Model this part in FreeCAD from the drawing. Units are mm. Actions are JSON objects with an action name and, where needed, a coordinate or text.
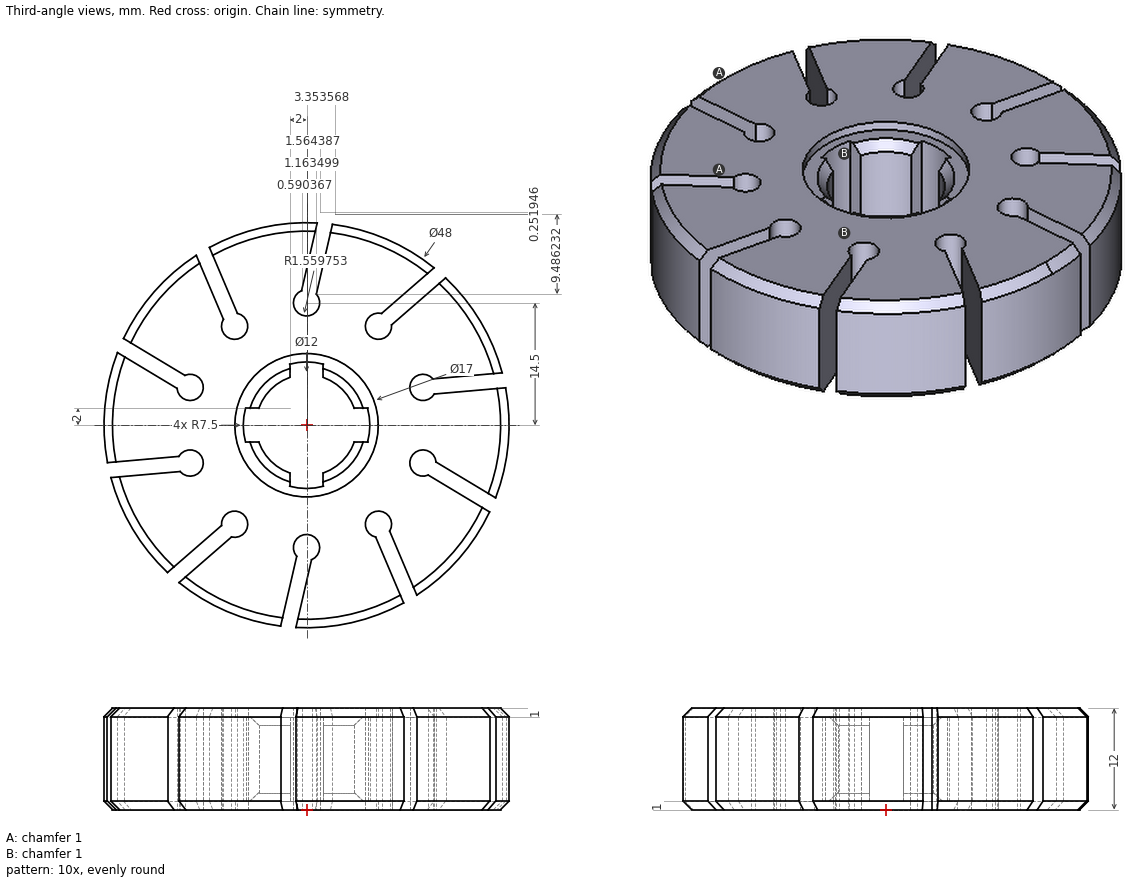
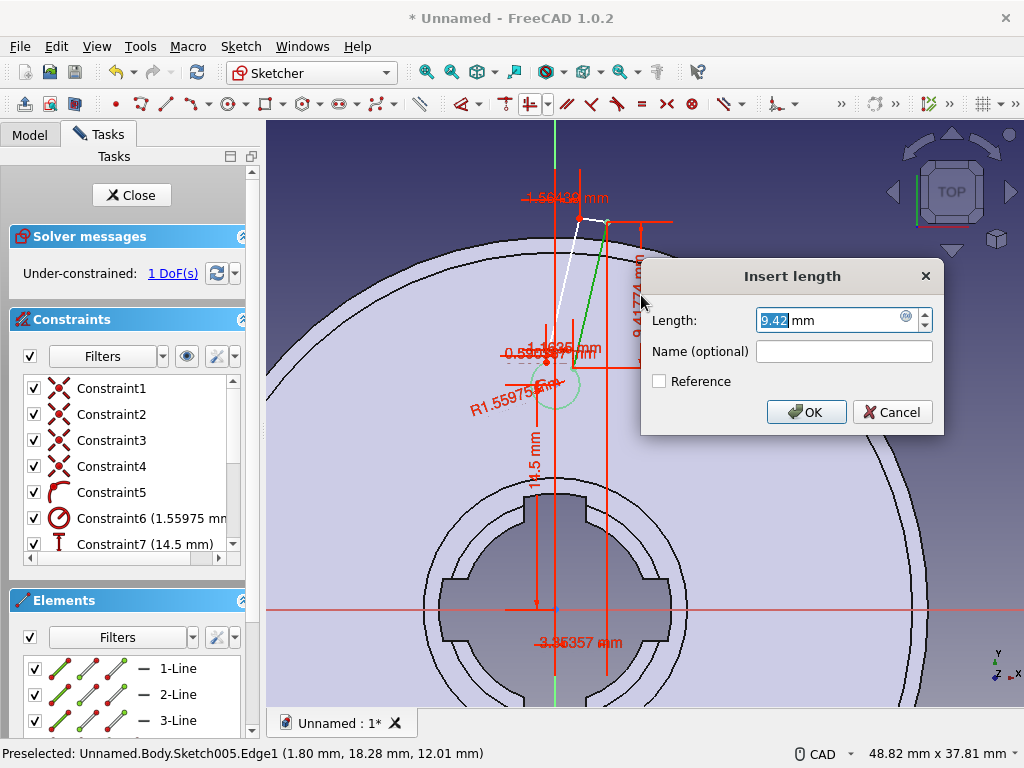
{"action": "type", "text": "9.486232"}
{"action": "key", "text": "Return"}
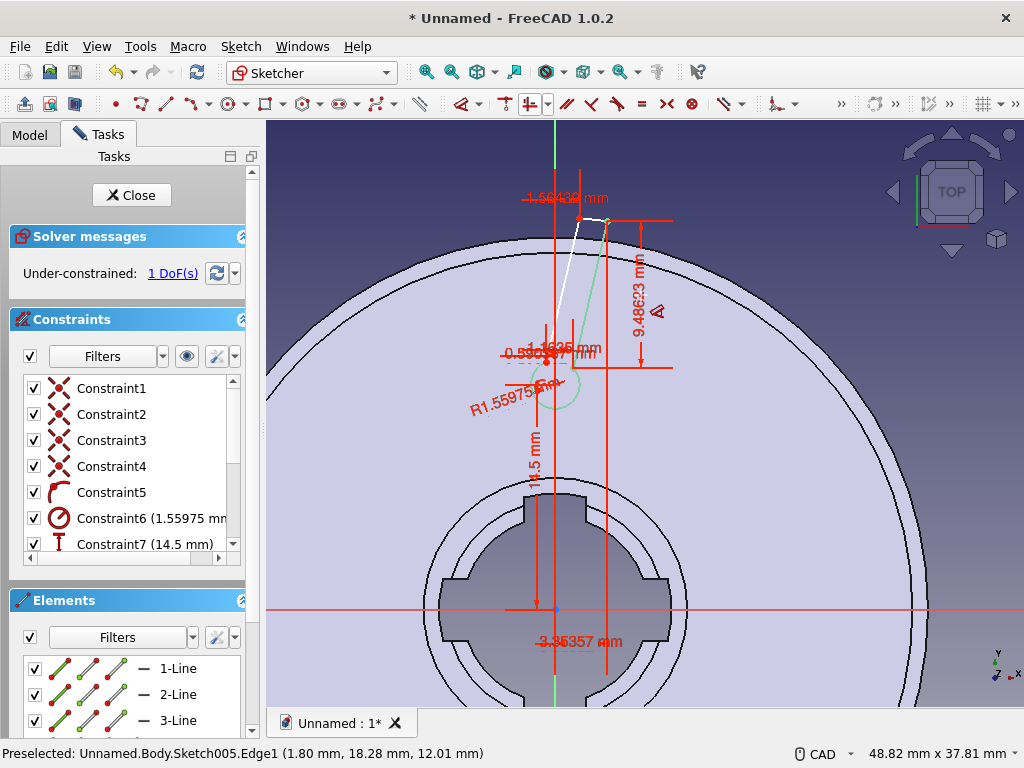
{"action": "scroll", "coordinate": [596, 220], "scroll_direction": "up", "scroll_amount": 12}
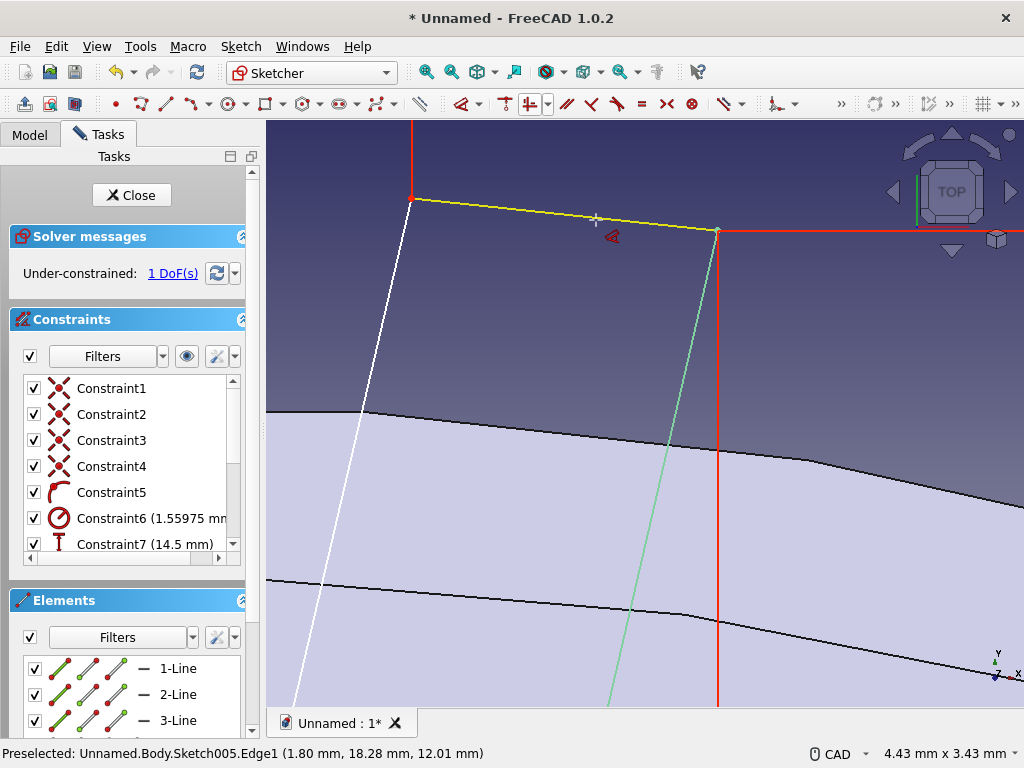
{"action": "left_click", "coordinate": [595, 218]}
{"action": "left_click", "coordinate": [752, 215]}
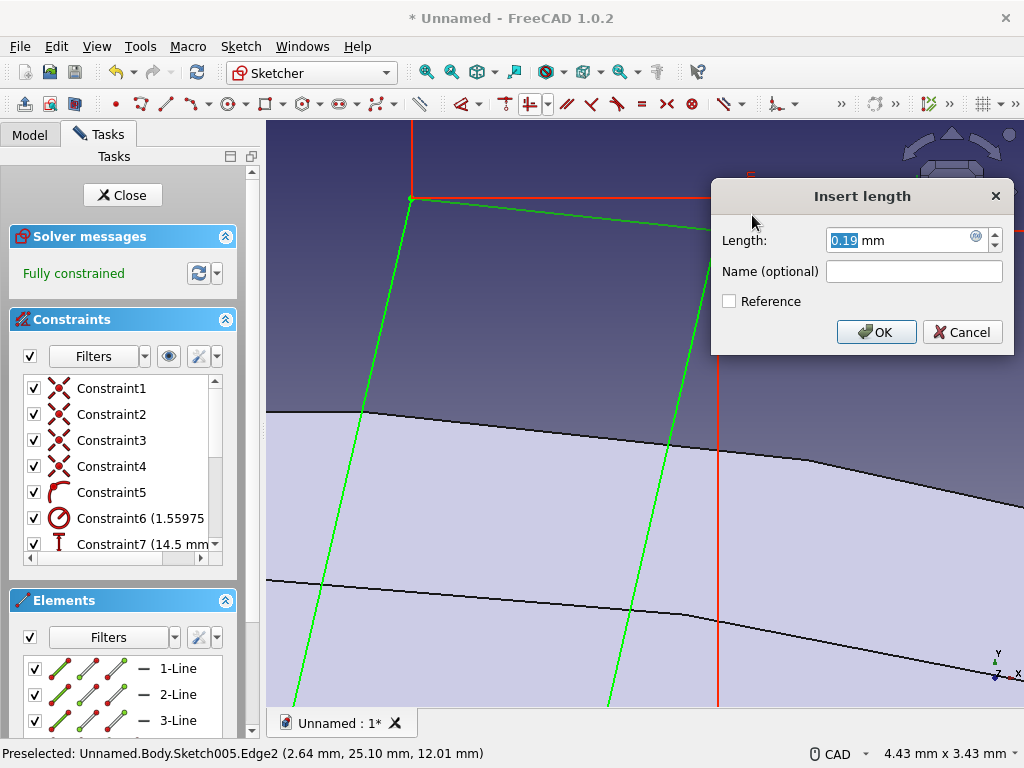
{"action": "type", "text": "0.251946"}
{"action": "key", "text": "Return"}
{"action": "key", "text": "Escape"}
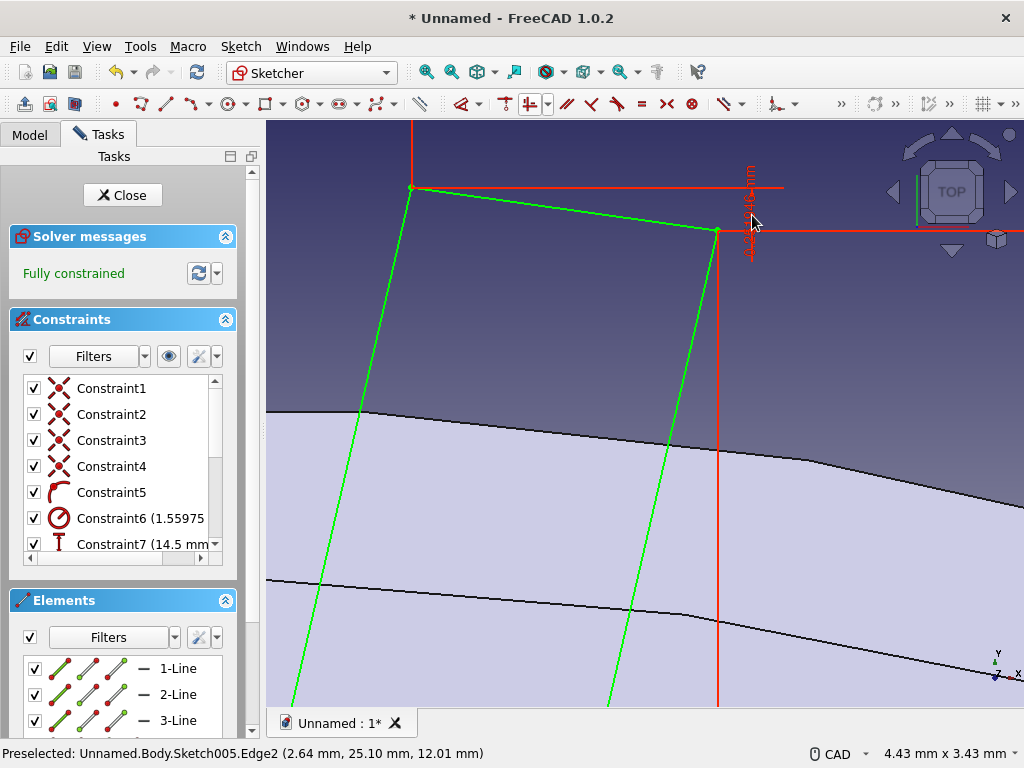
{"action": "left_click", "coordinate": [123, 195]}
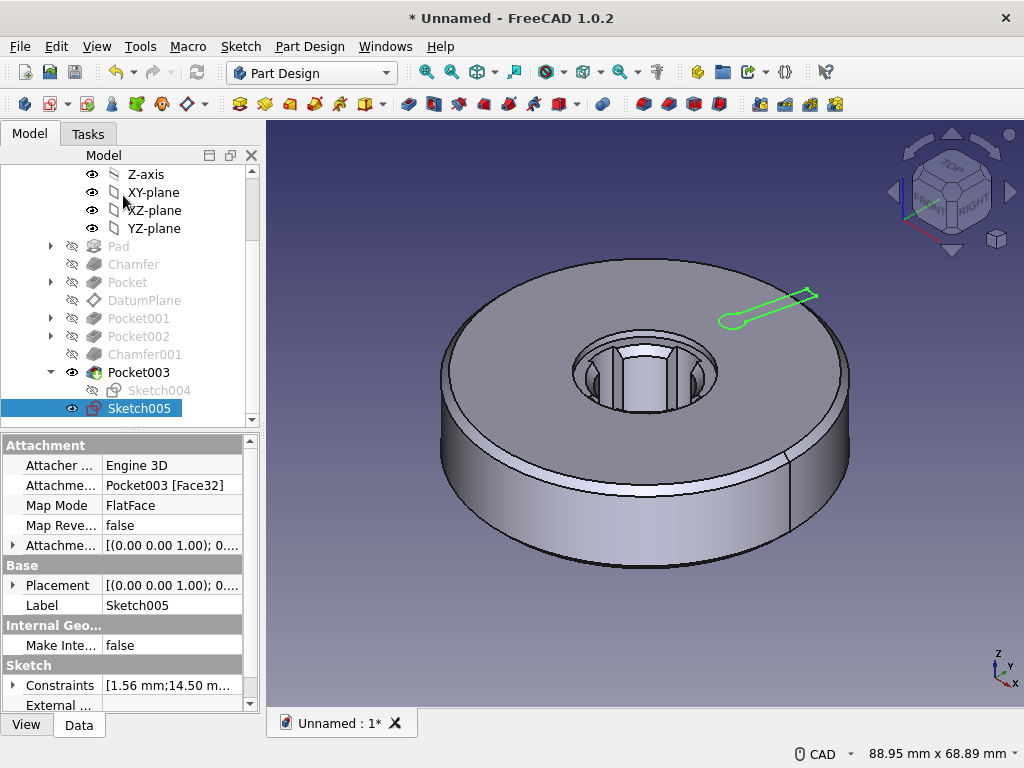
{"action": "left_click", "coordinate": [409, 104]}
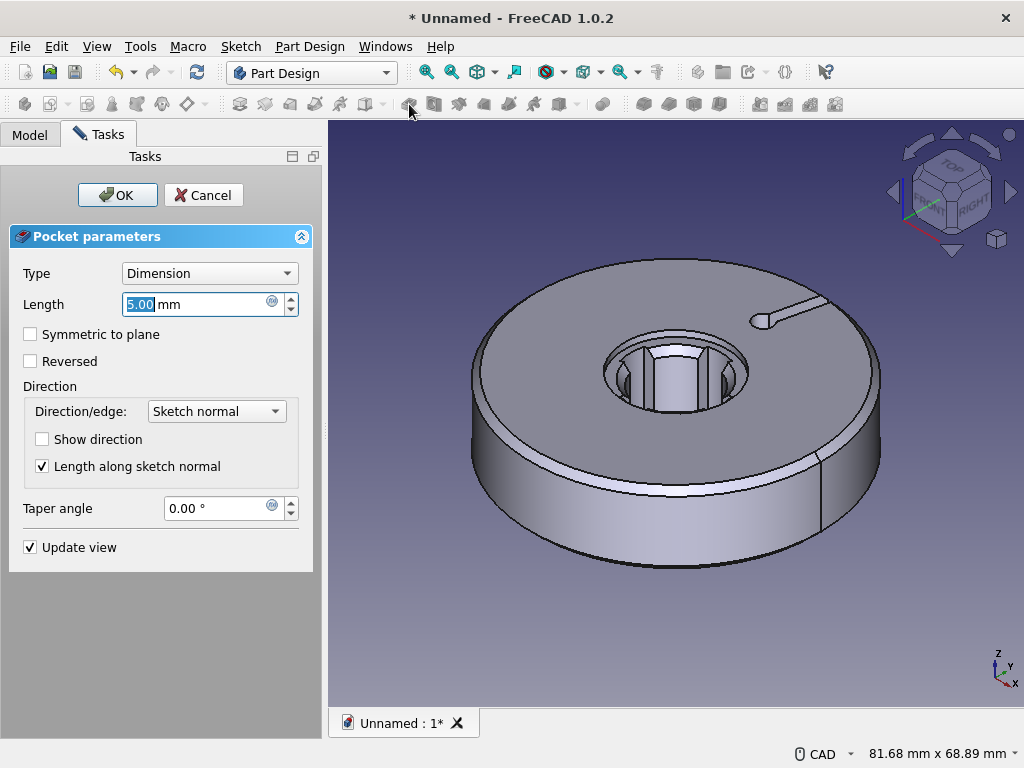
{"action": "left_click", "coordinate": [210, 274]}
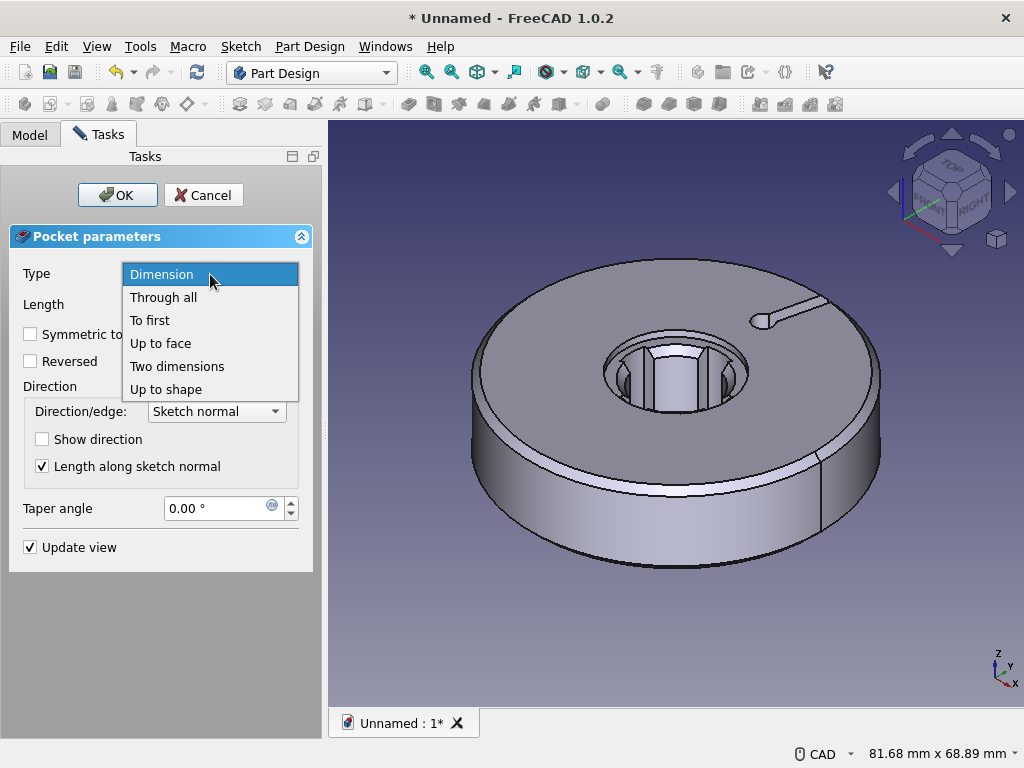
{"action": "left_click", "coordinate": [208, 298]}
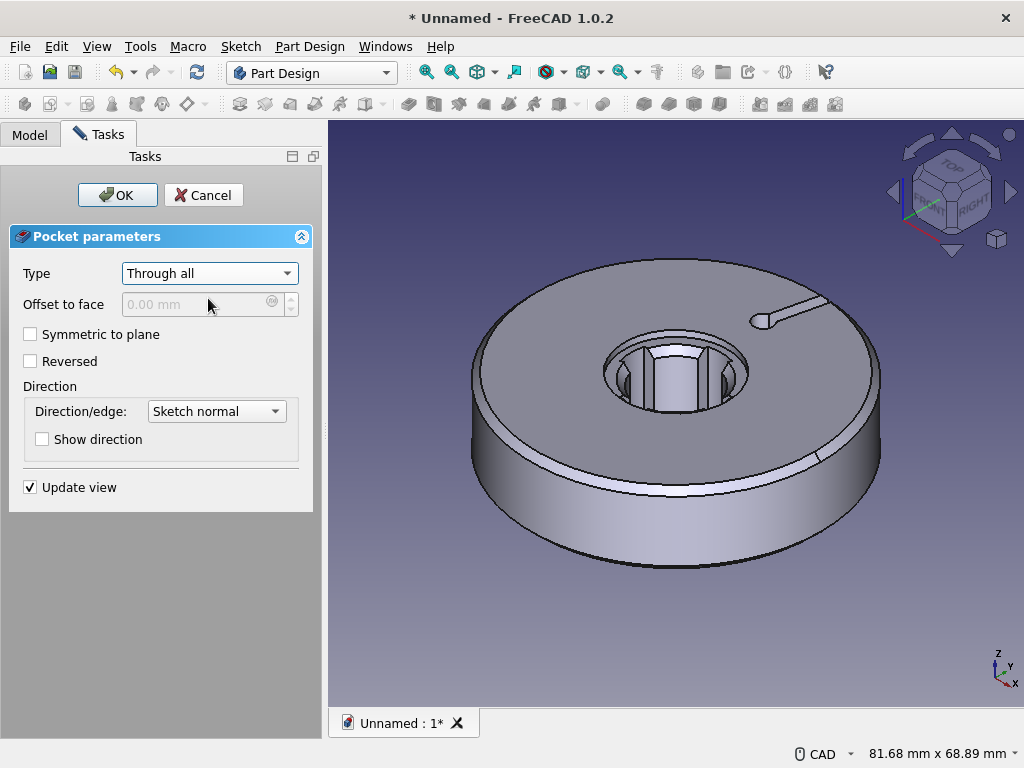
{"action": "left_click", "coordinate": [118, 195]}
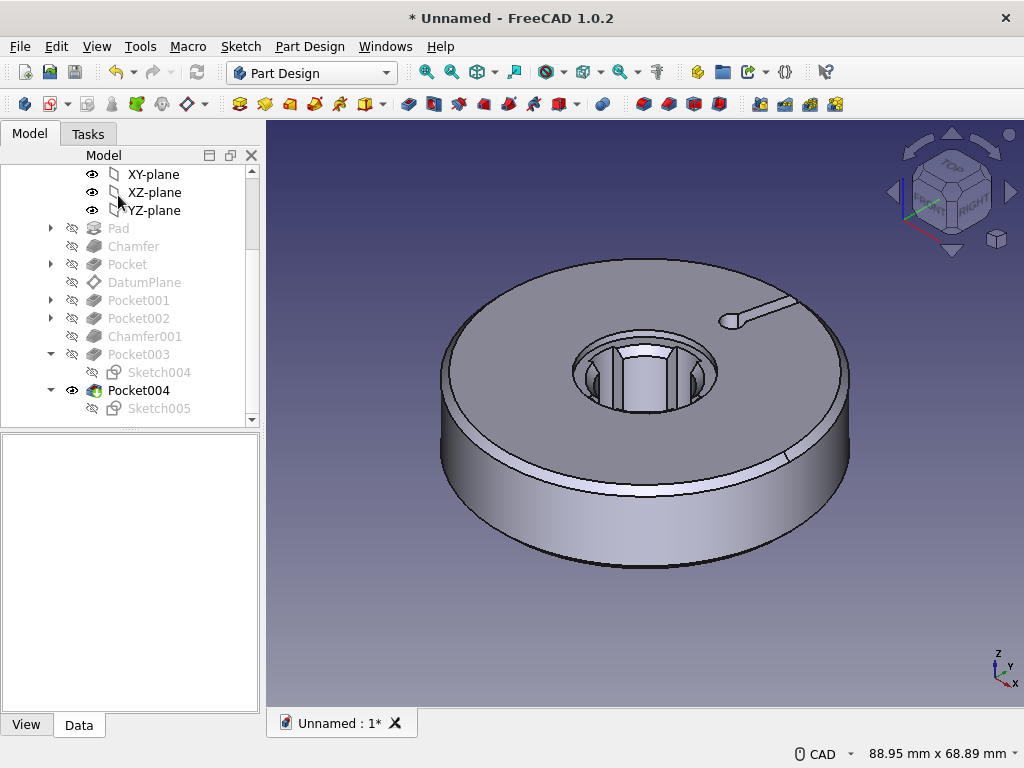
{"action": "left_click", "coordinate": [117, 390]}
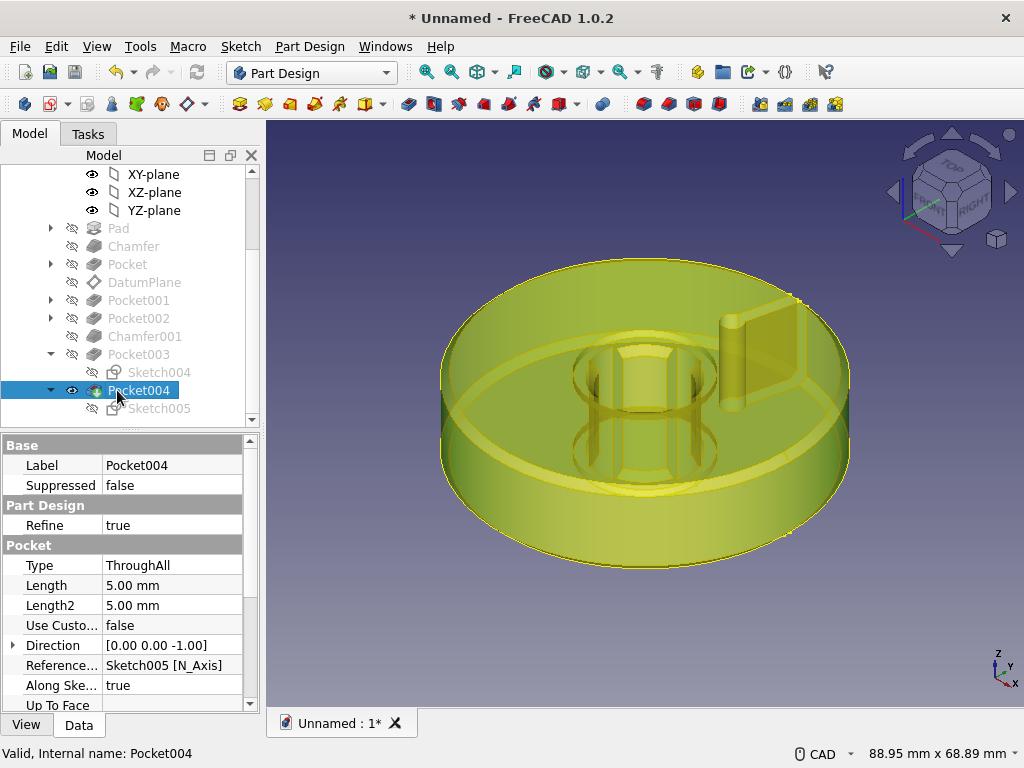
{"action": "left_click", "coordinate": [810, 104]}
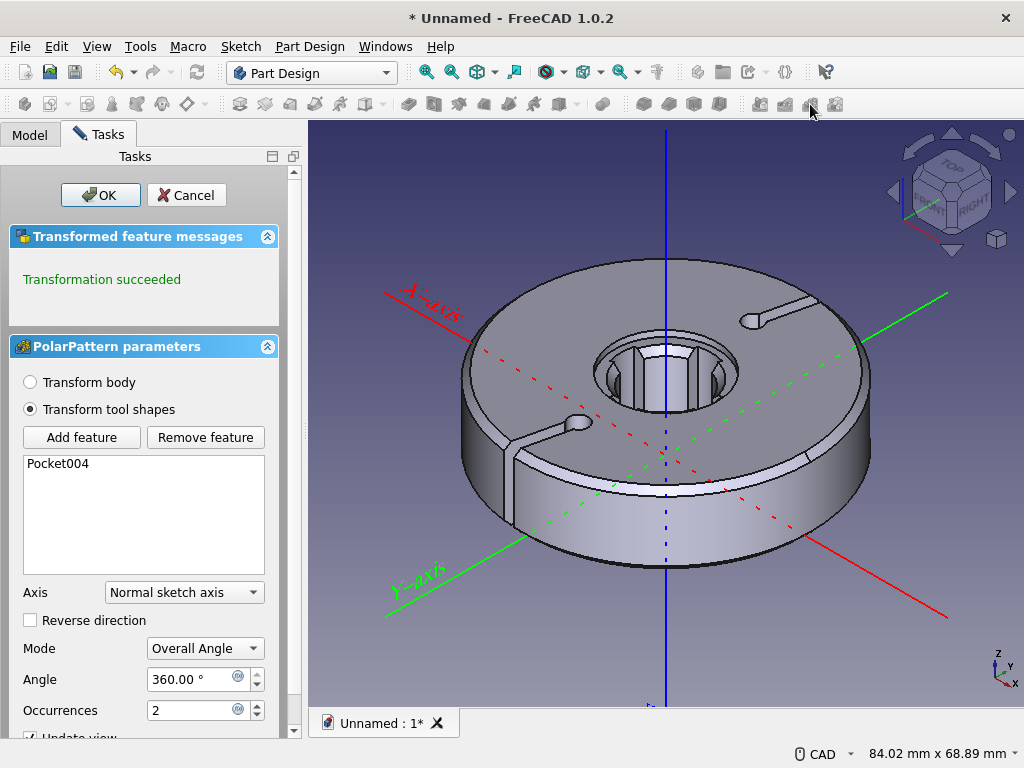
{"action": "left_click", "coordinate": [185, 592]}